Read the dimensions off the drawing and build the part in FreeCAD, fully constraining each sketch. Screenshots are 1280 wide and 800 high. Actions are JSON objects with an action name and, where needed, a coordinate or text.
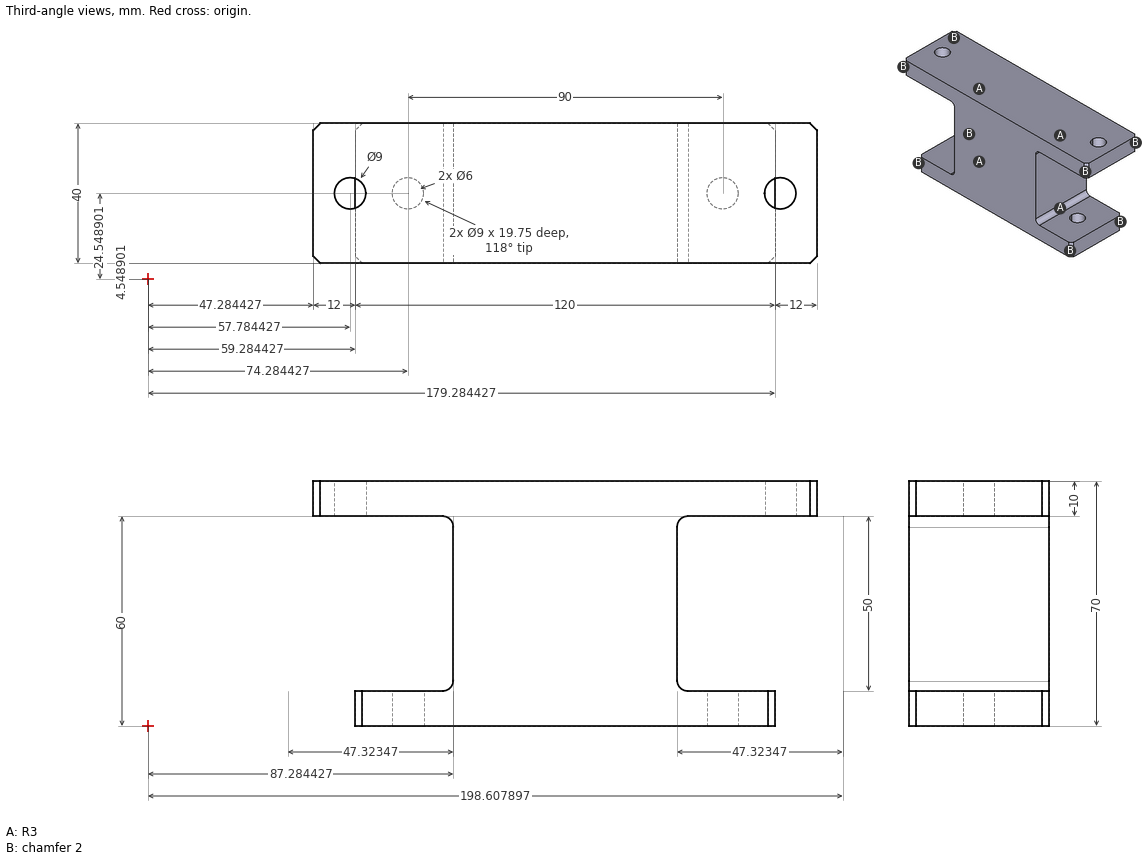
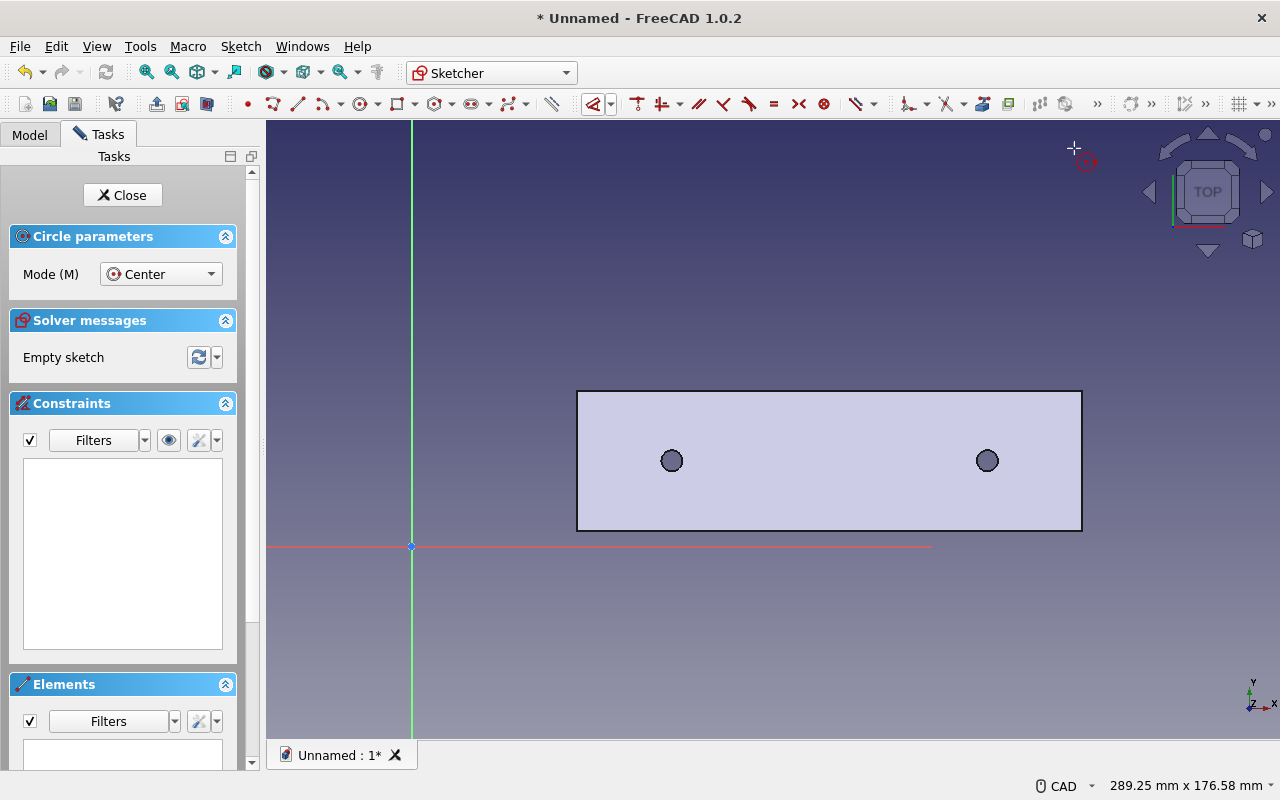
{"action": "scroll", "coordinate": [672, 461], "scroll_direction": "up", "scroll_amount": 4}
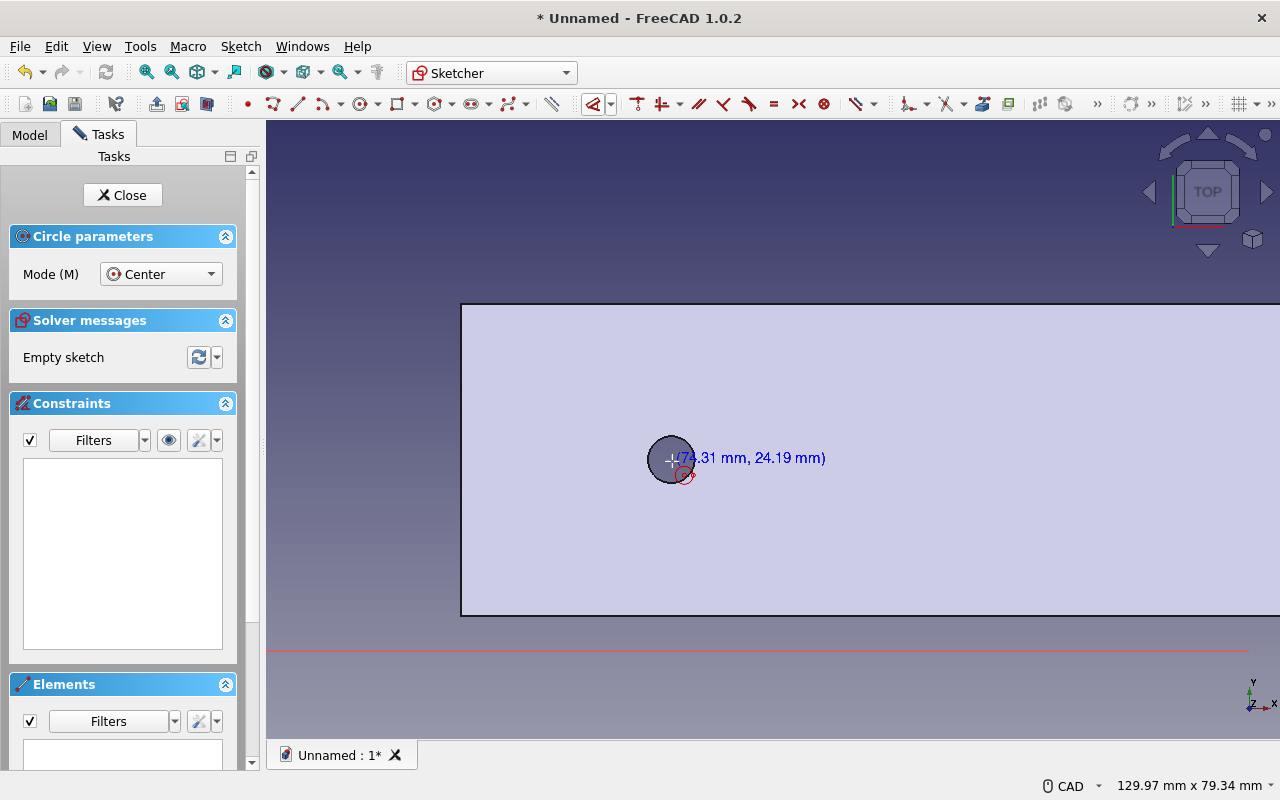
{"action": "left_click", "coordinate": [671, 460]}
{"action": "left_click", "coordinate": [688, 443]}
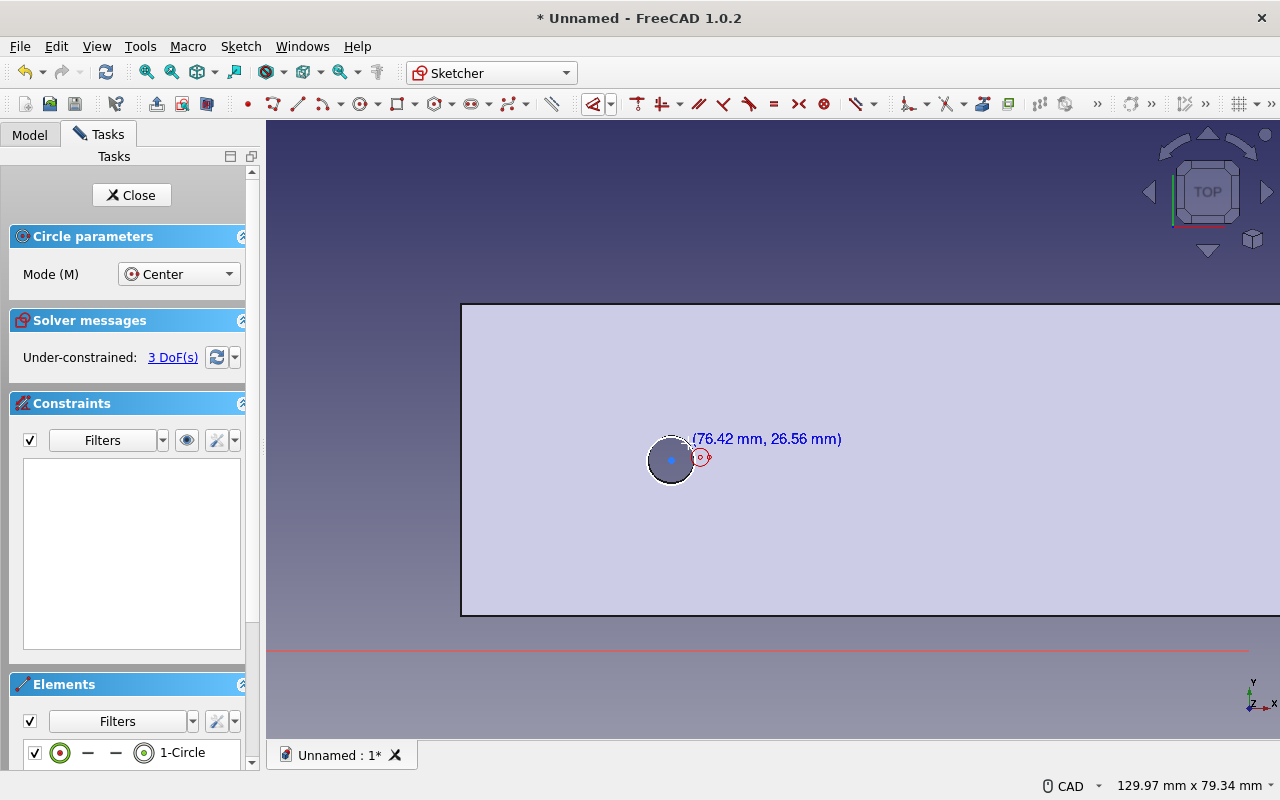
{"action": "scroll", "coordinate": [672, 336], "scroll_direction": "down", "scroll_amount": 4}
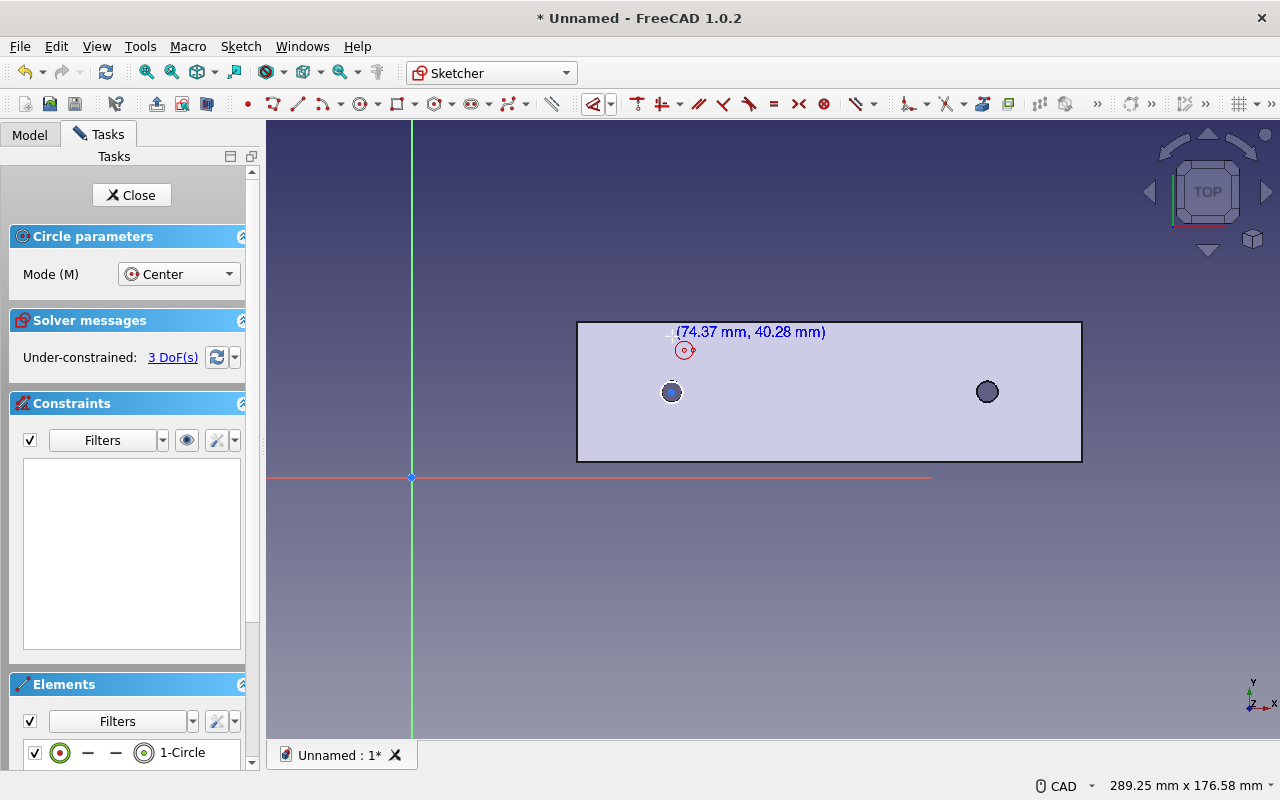
{"action": "scroll", "coordinate": [987, 392], "scroll_direction": "up", "scroll_amount": 4}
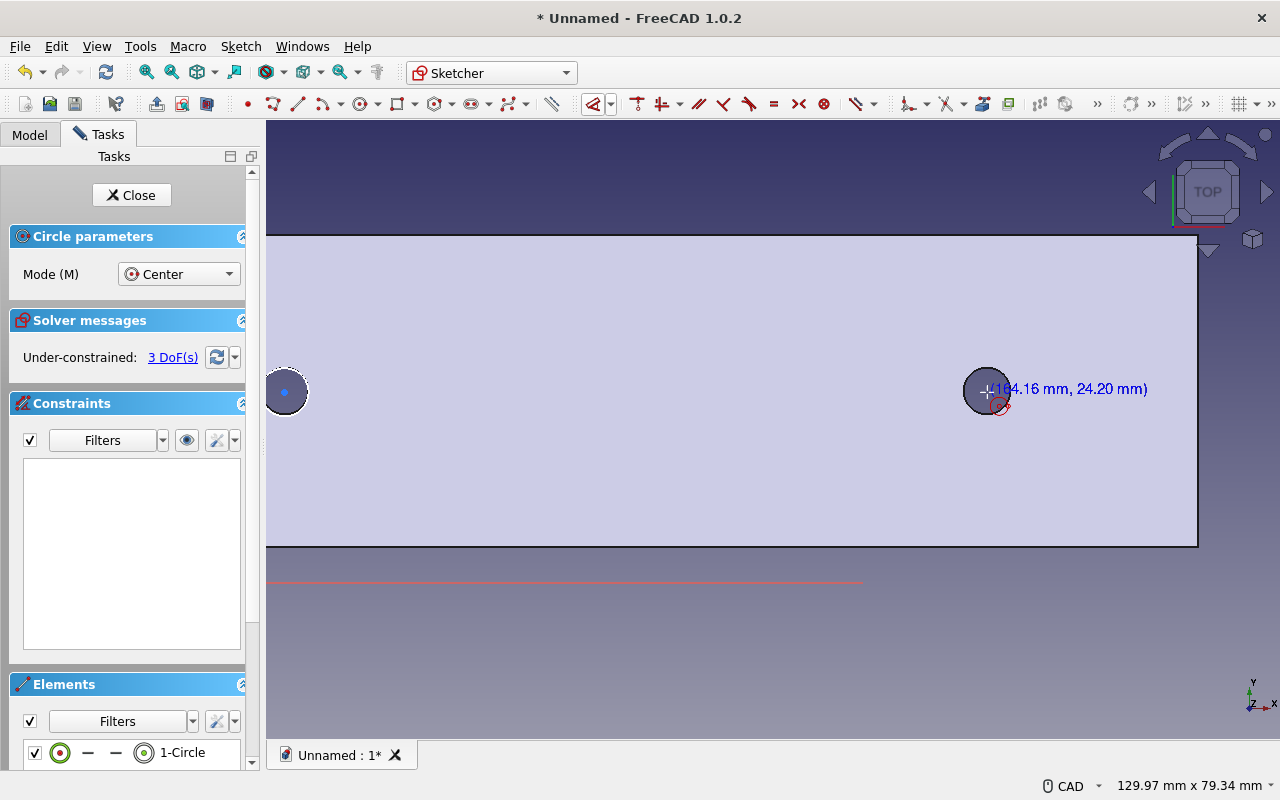
{"action": "left_click", "coordinate": [987, 391]}
{"action": "left_click", "coordinate": [1004, 374]}
{"action": "key", "text": "Escape"}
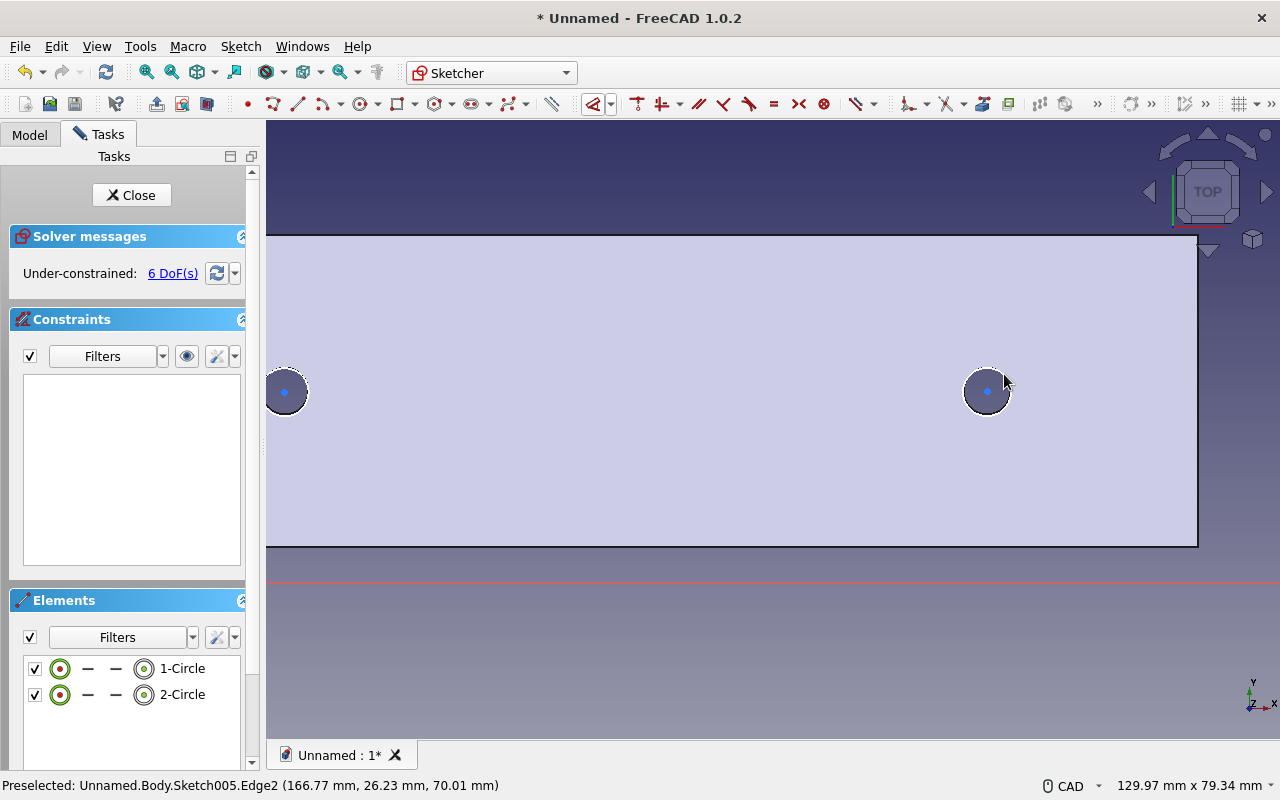
{"action": "left_click", "coordinate": [302, 375]}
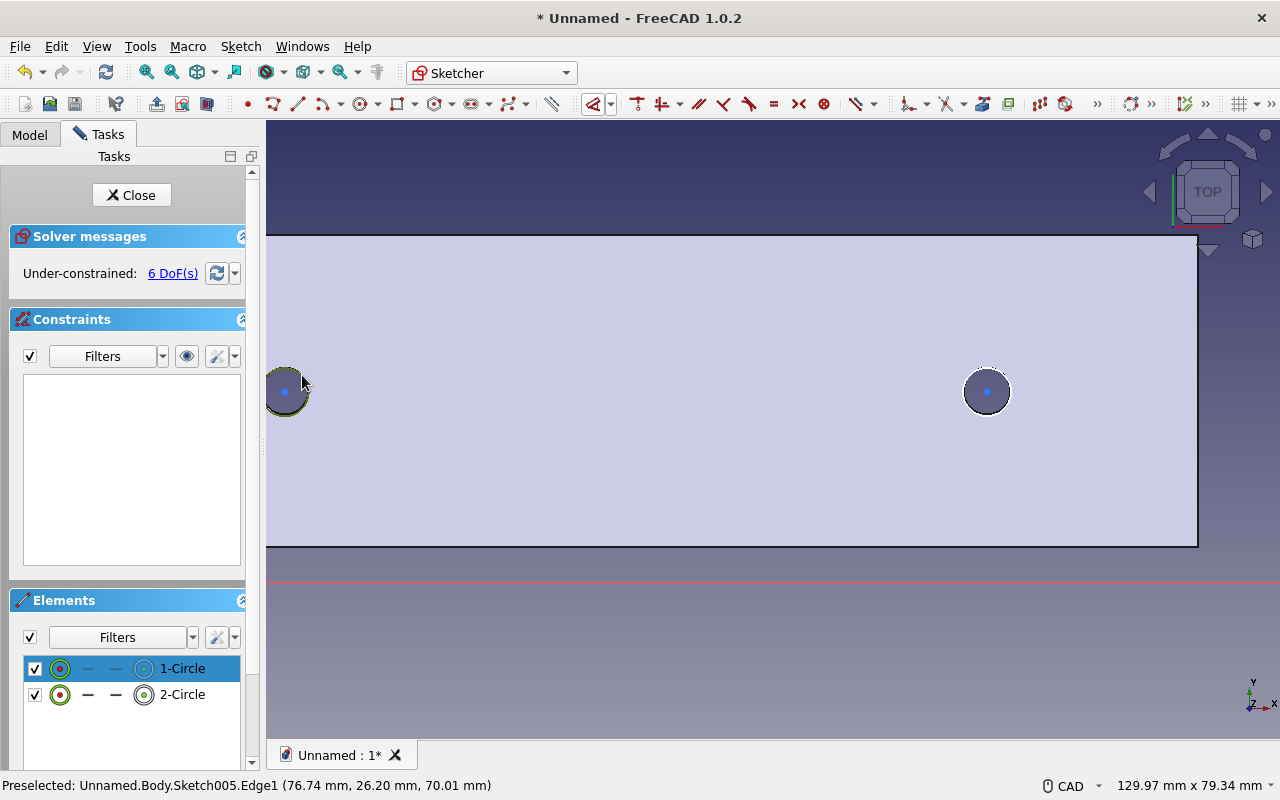
{"action": "left_click", "coordinate": [1004, 375]}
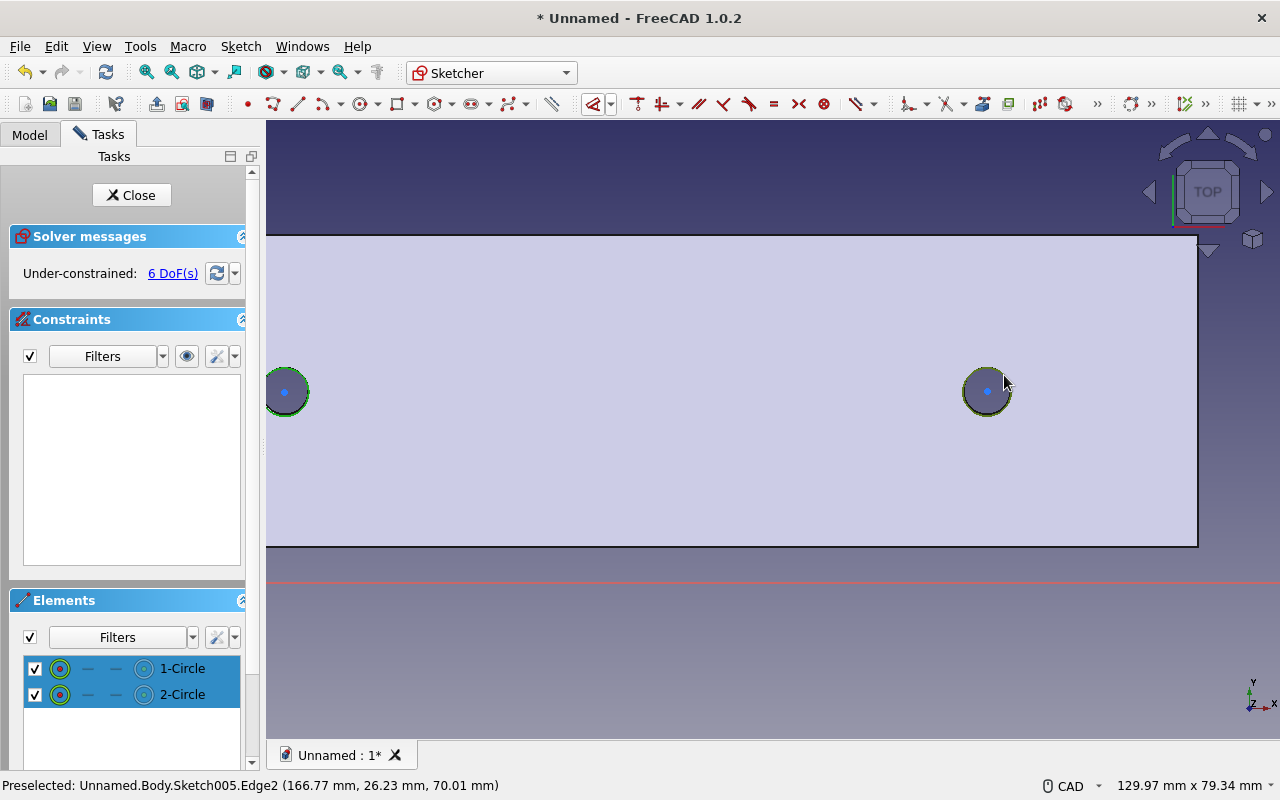
{"action": "left_click", "coordinate": [774, 104]}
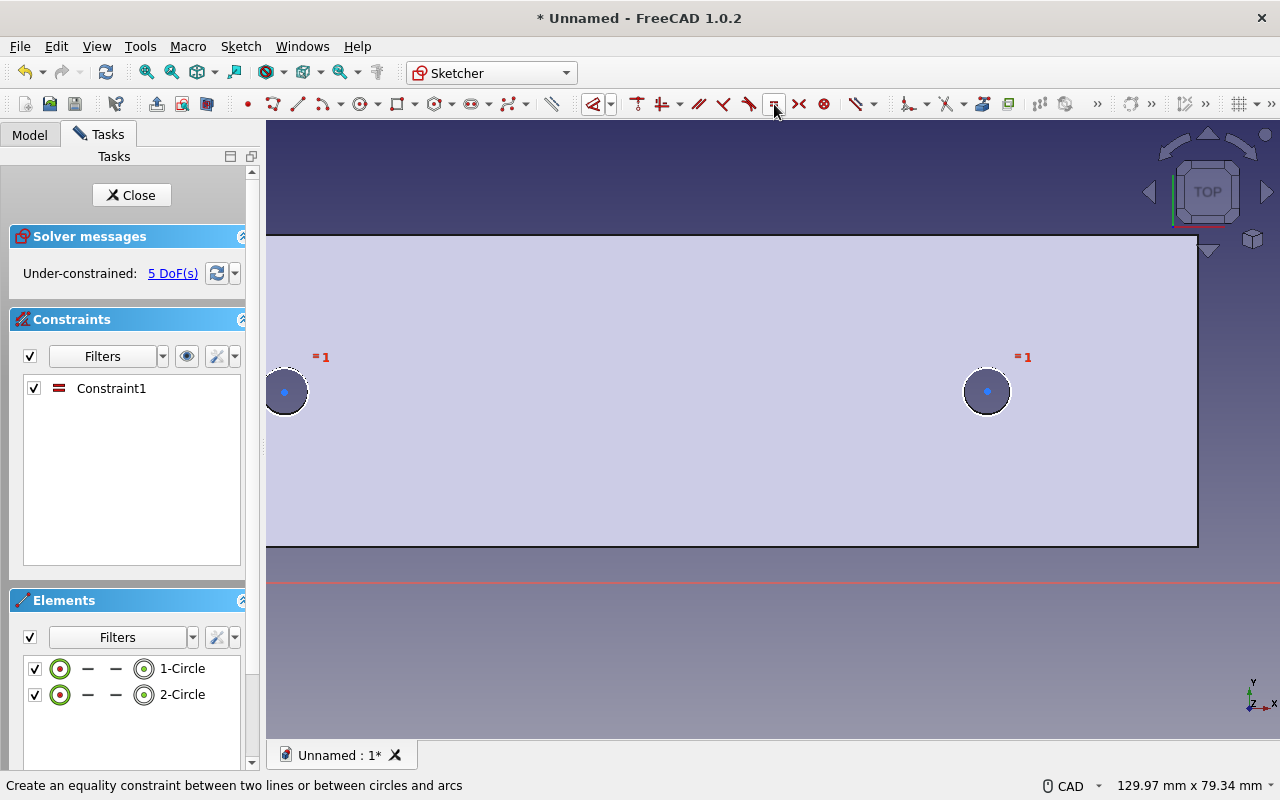
{"action": "scroll", "coordinate": [987, 392], "scroll_direction": "down", "scroll_amount": 4}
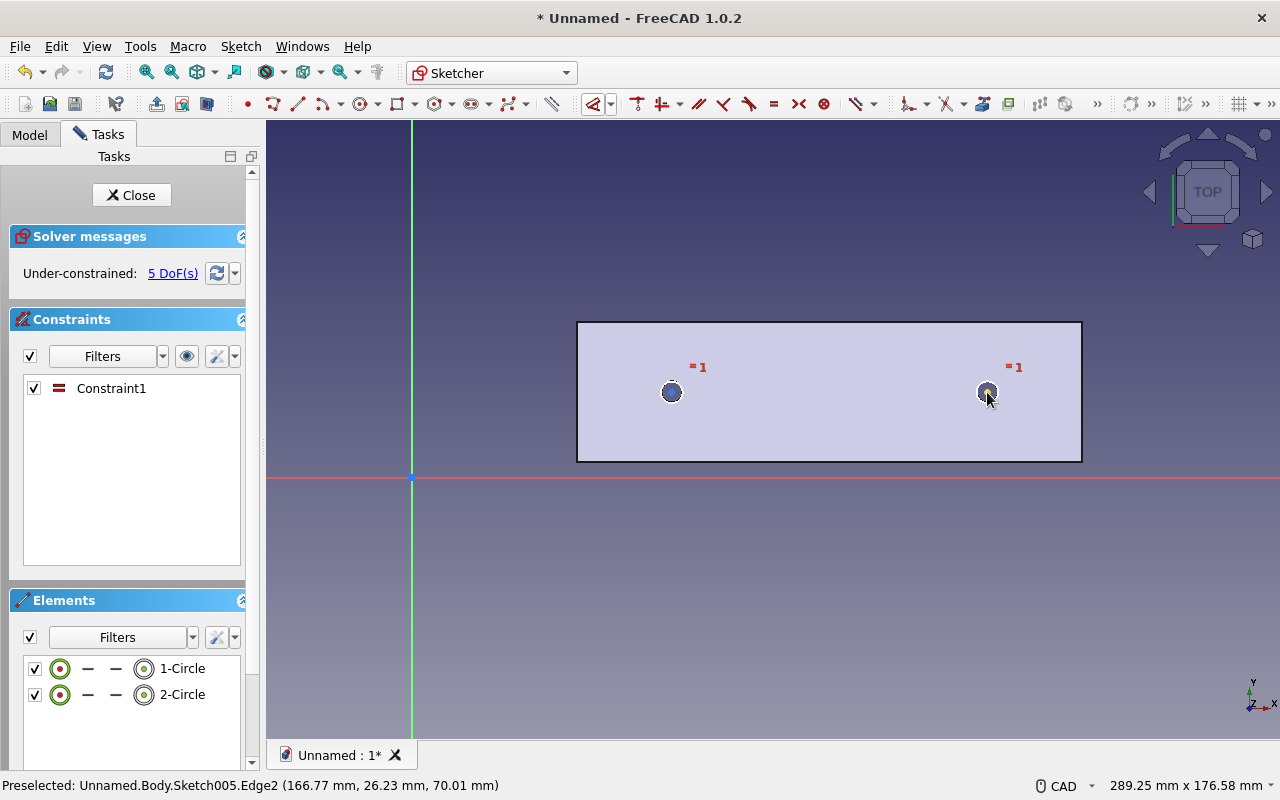
{"action": "left_click", "coordinate": [672, 392]}